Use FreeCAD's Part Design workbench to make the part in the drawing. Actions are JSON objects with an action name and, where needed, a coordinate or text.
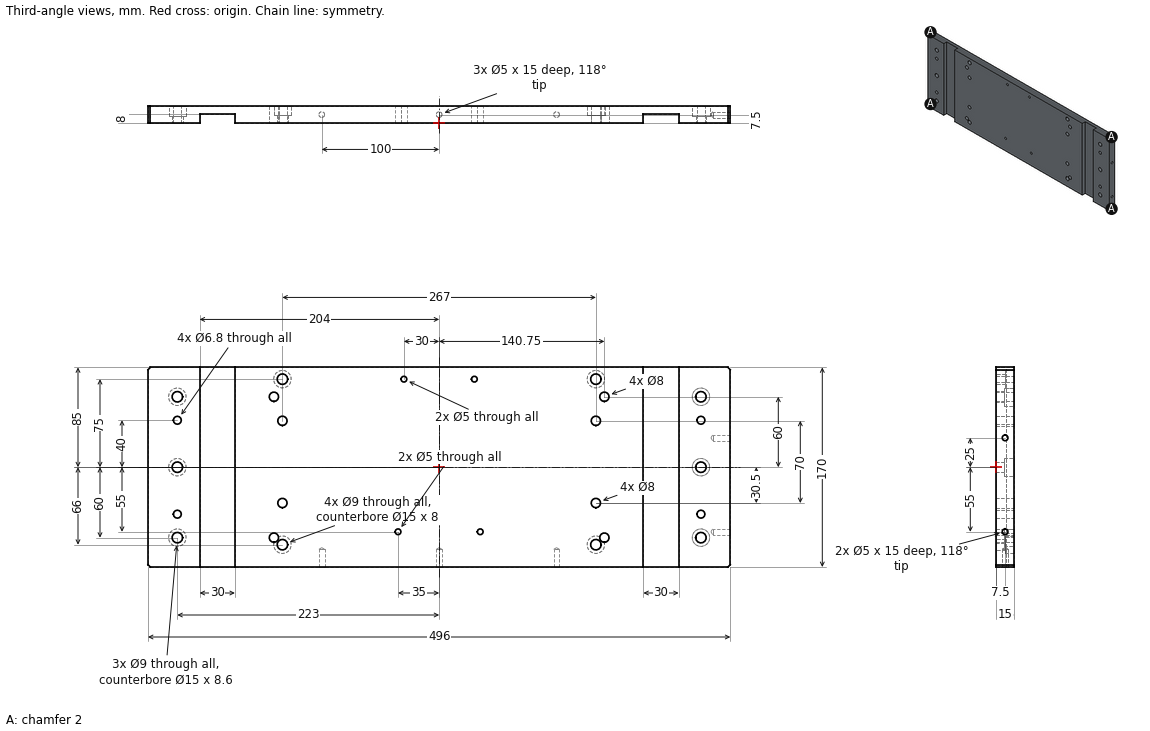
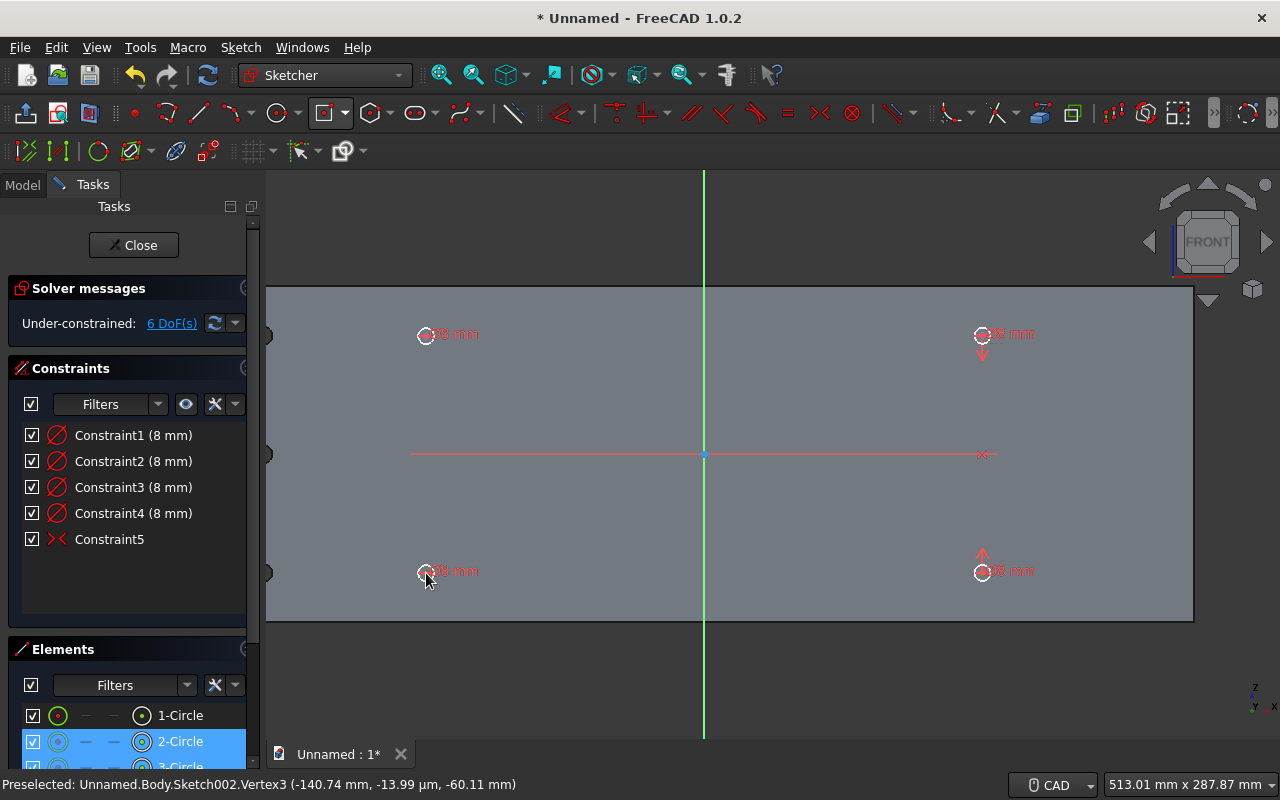
{"action": "left_click", "coordinate": [704, 674]}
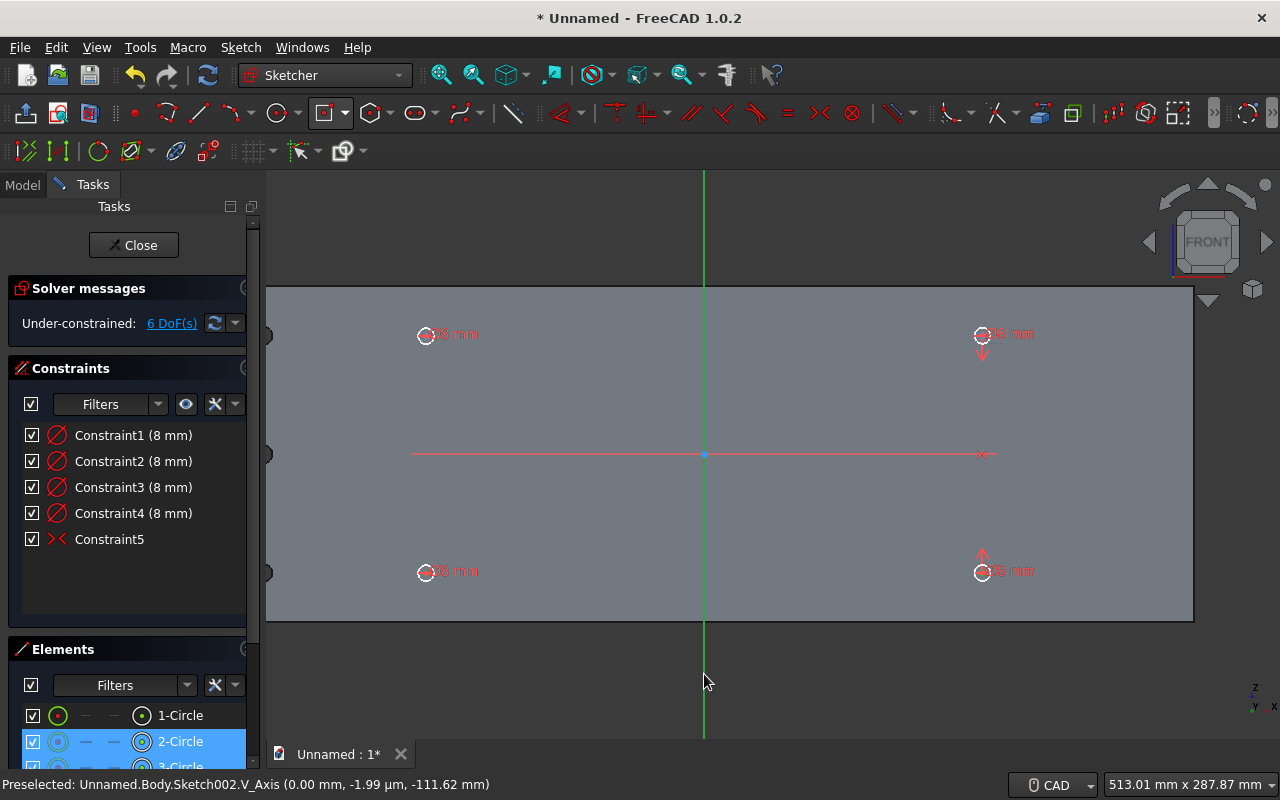
{"action": "left_click", "coordinate": [820, 114]}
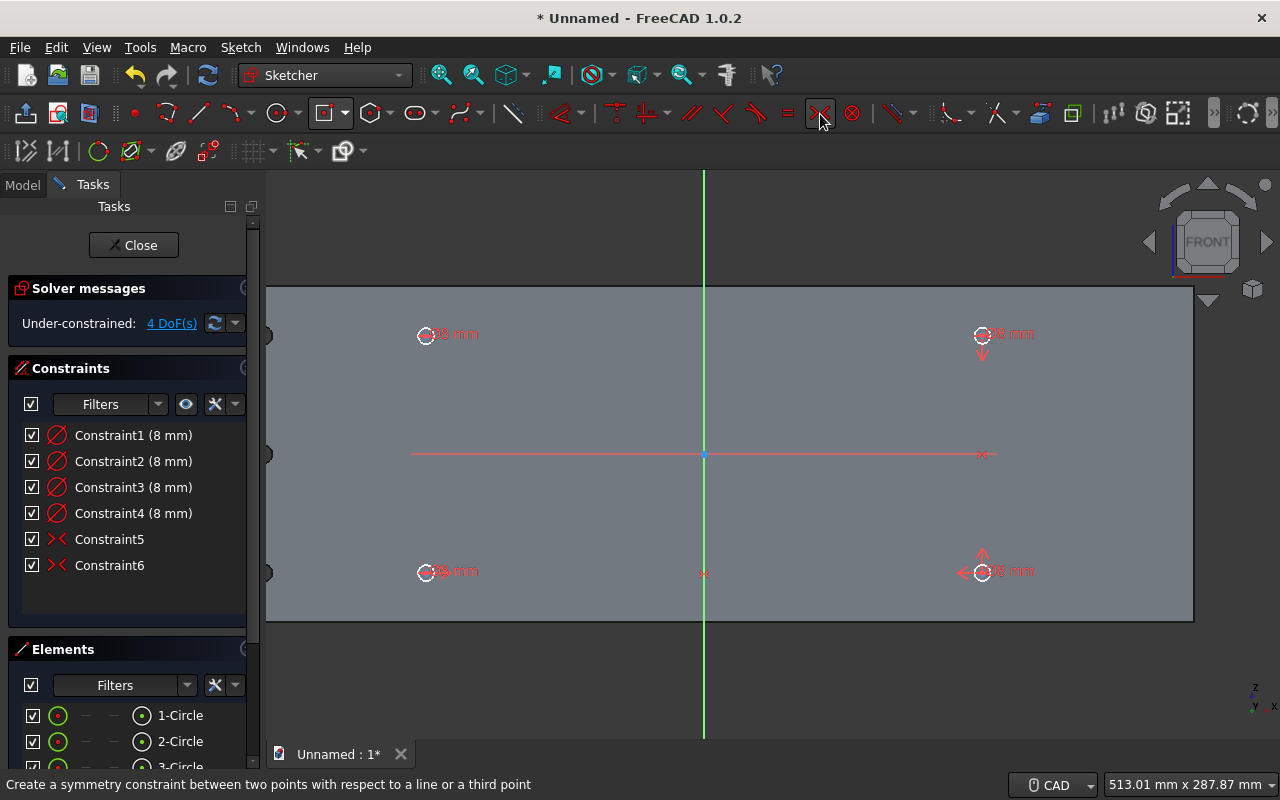
{"action": "left_click", "coordinate": [982, 336]}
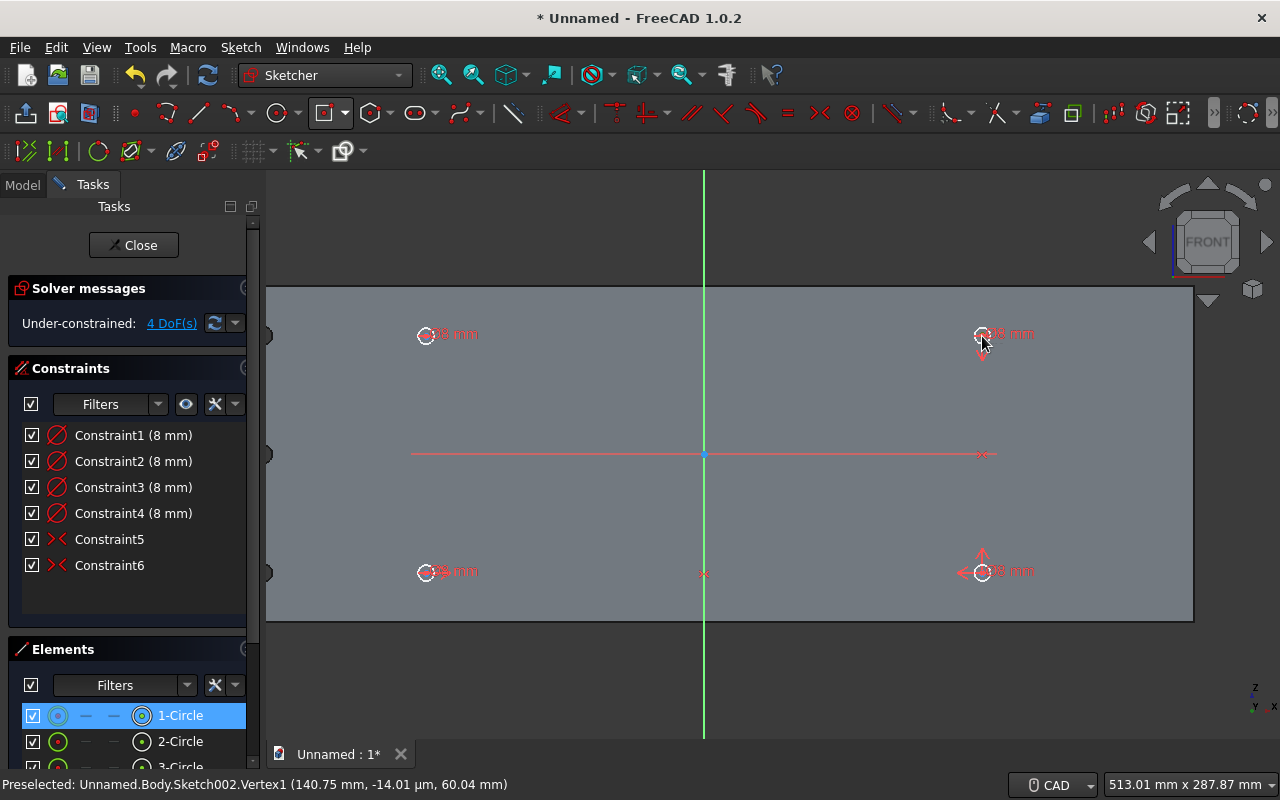
{"action": "left_click", "coordinate": [426, 336]}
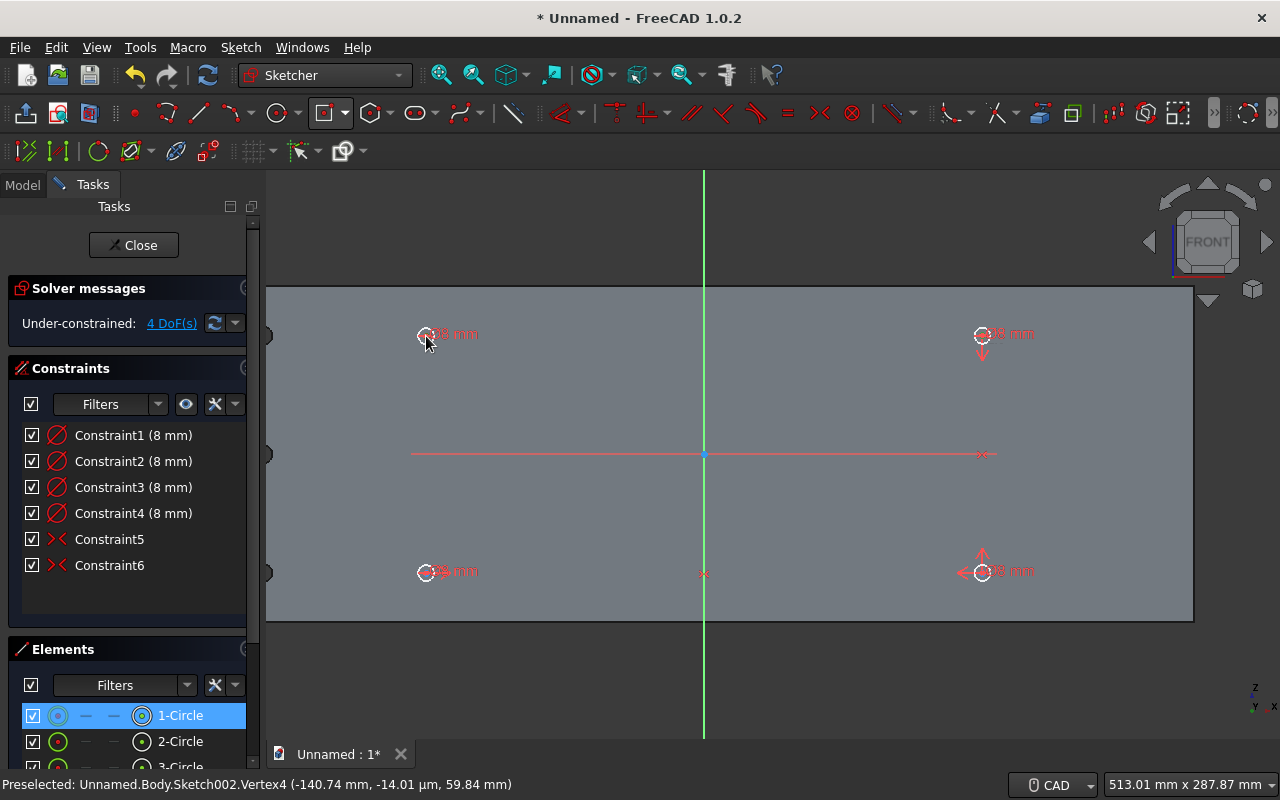
{"action": "left_click", "coordinate": [704, 674]}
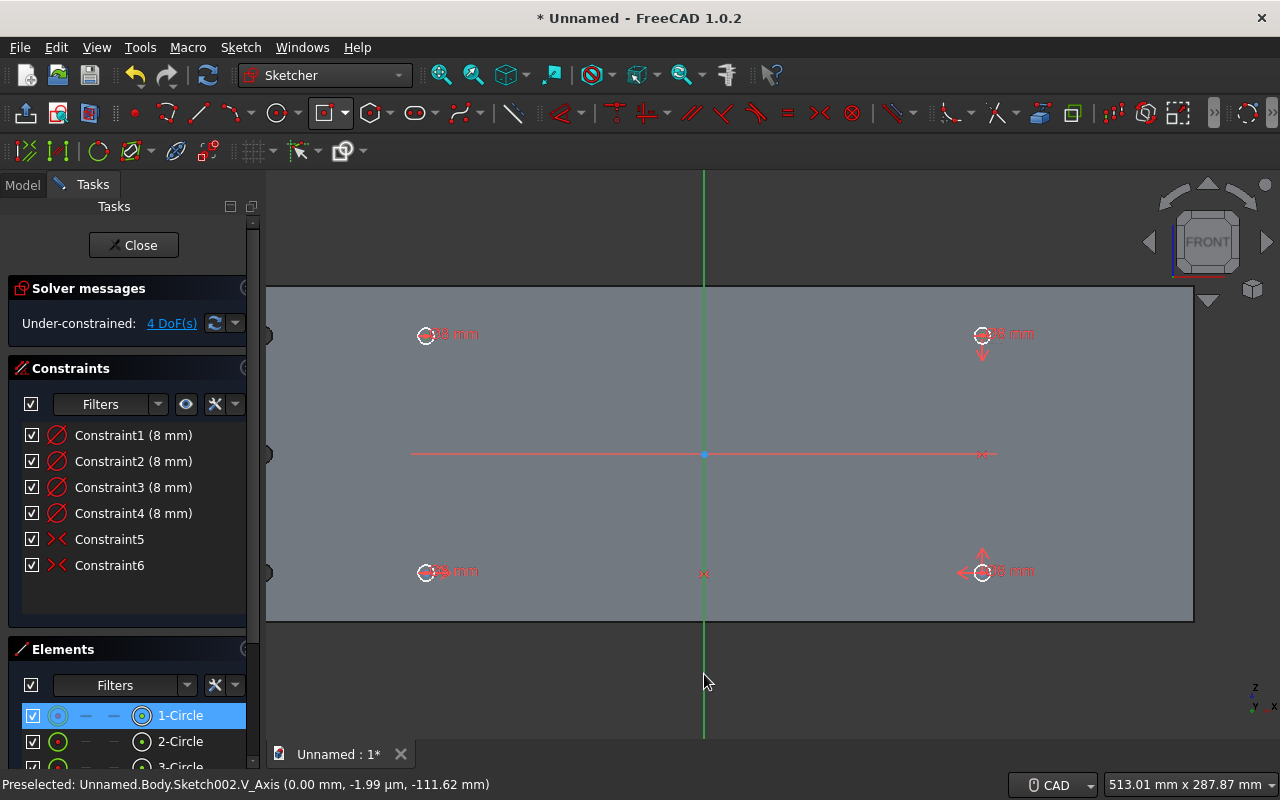
{"action": "left_click", "coordinate": [820, 114]}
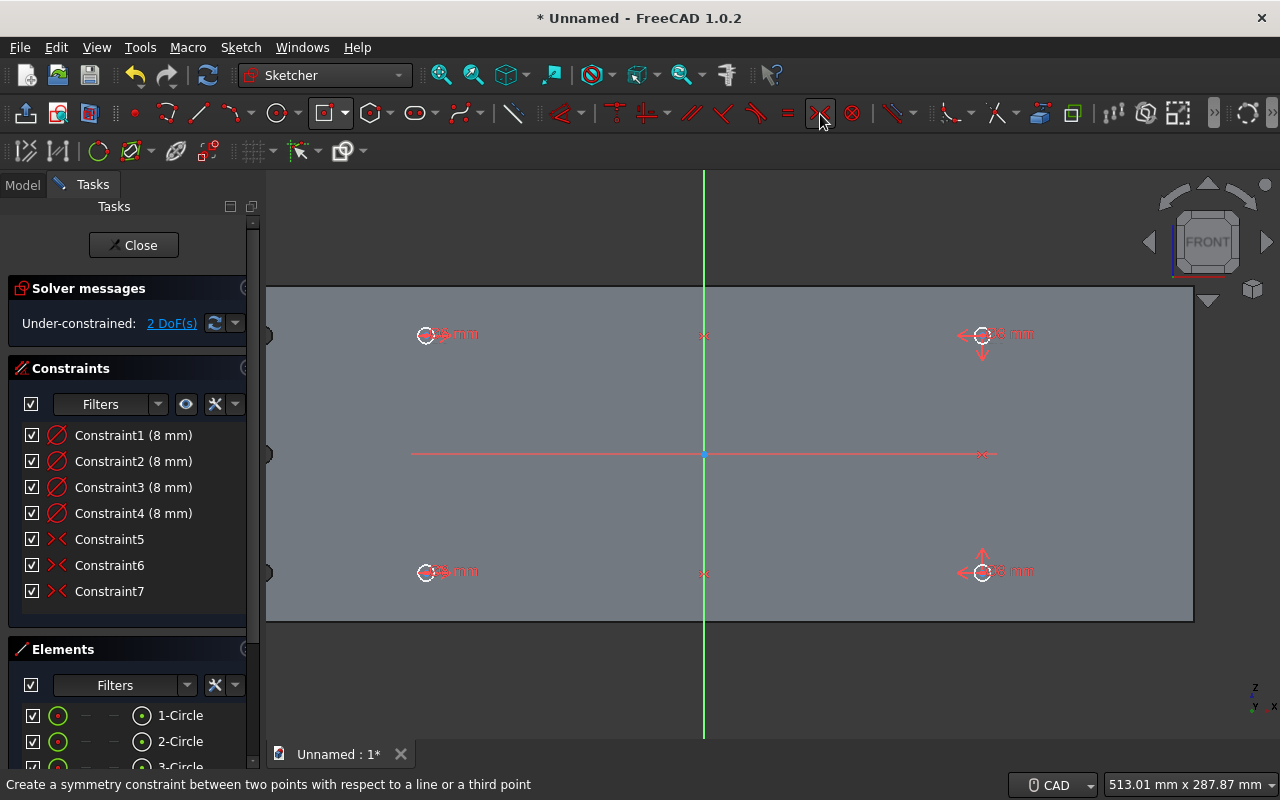
{"action": "left_click", "coordinate": [560, 114]}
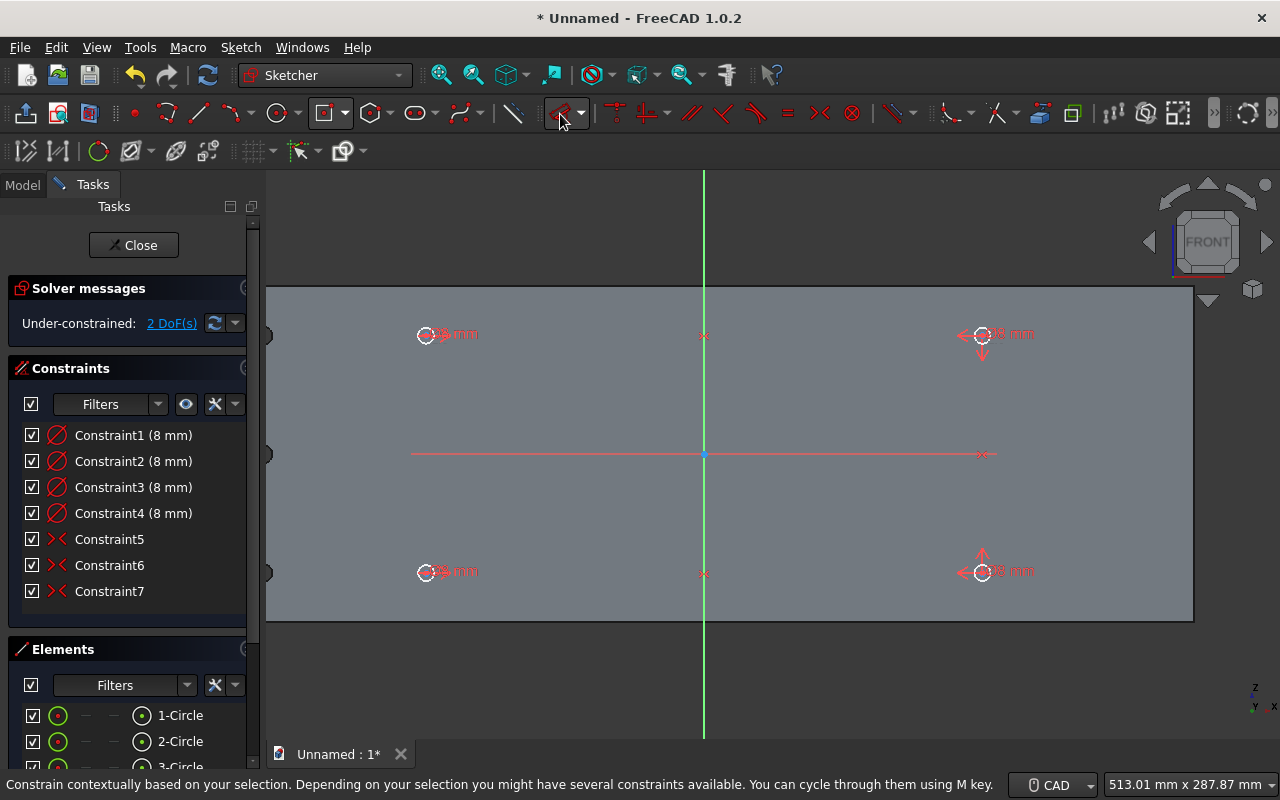
{"action": "left_click", "coordinate": [982, 336]}
{"action": "left_click", "coordinate": [1016, 395]}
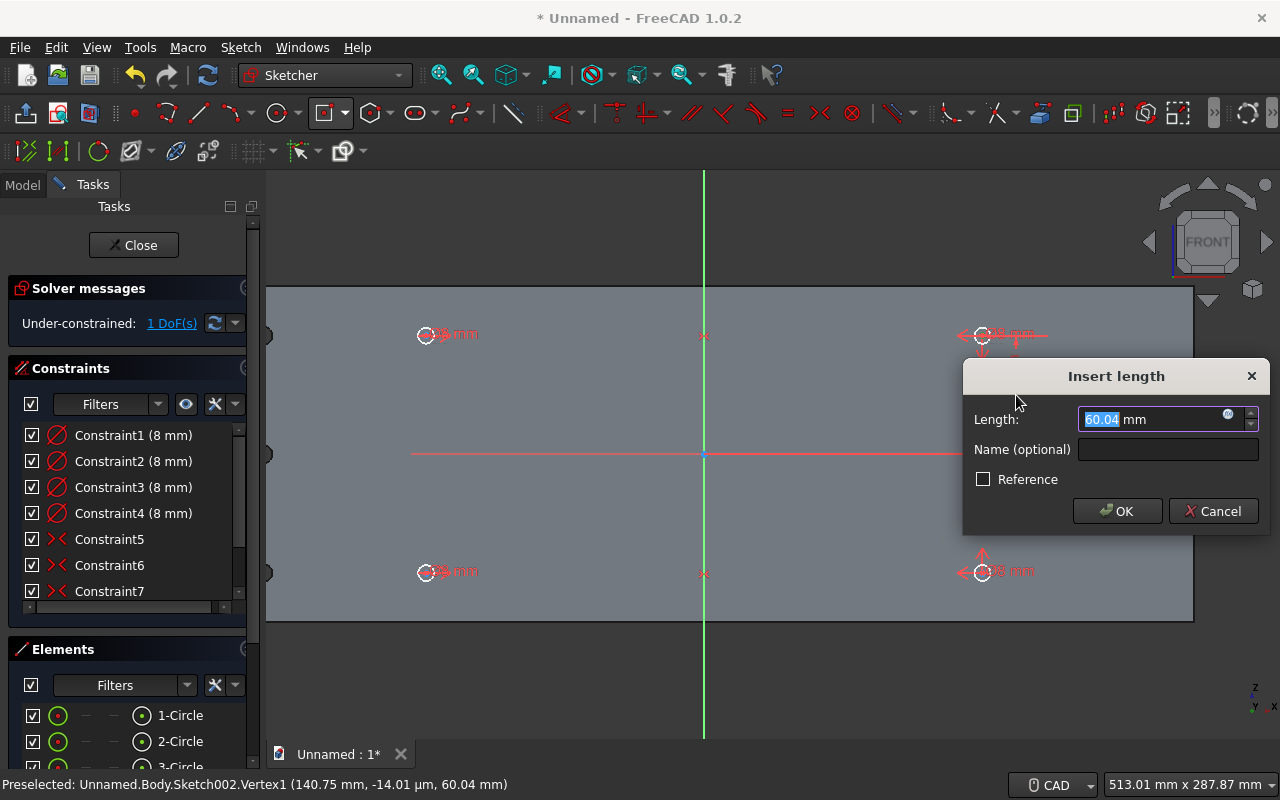
{"action": "type", "text": "60"}
{"action": "key", "text": "Return"}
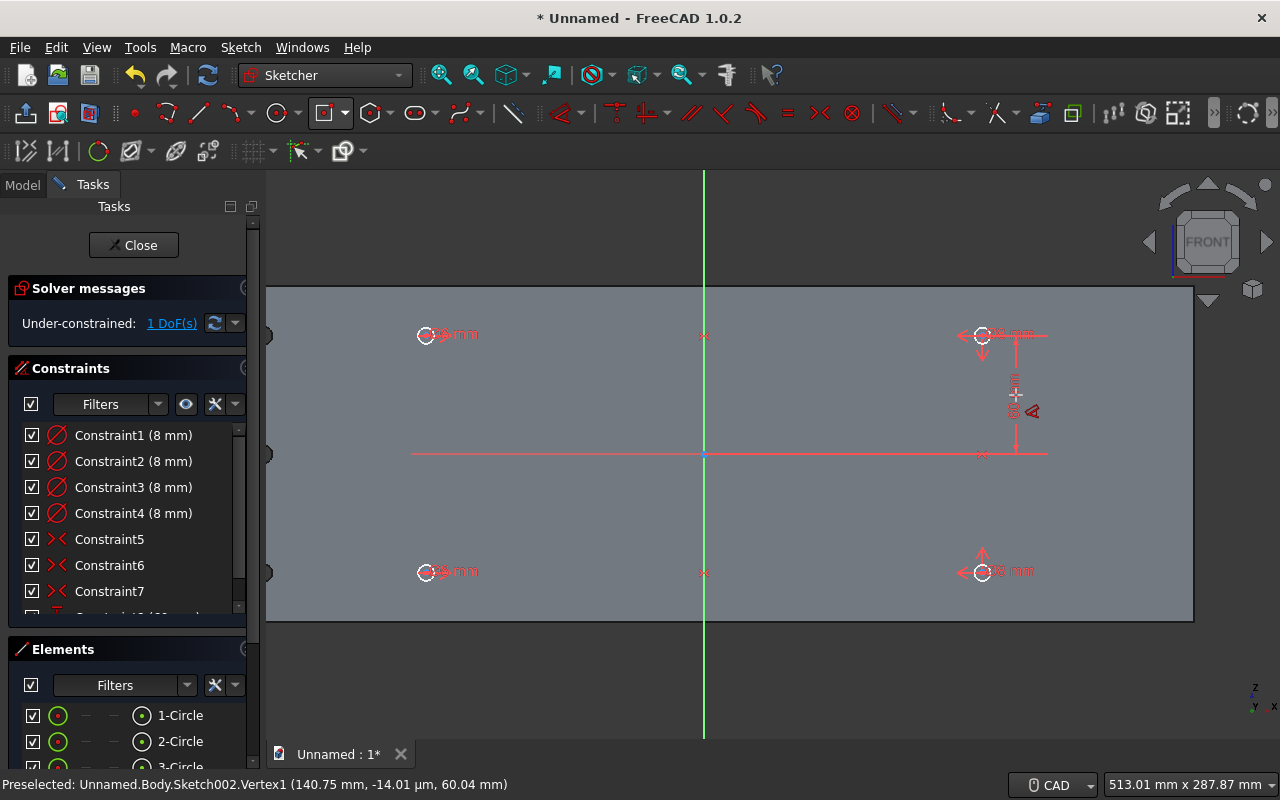
{"action": "left_click", "coordinate": [982, 336]}
{"action": "left_click", "coordinate": [843, 302]}